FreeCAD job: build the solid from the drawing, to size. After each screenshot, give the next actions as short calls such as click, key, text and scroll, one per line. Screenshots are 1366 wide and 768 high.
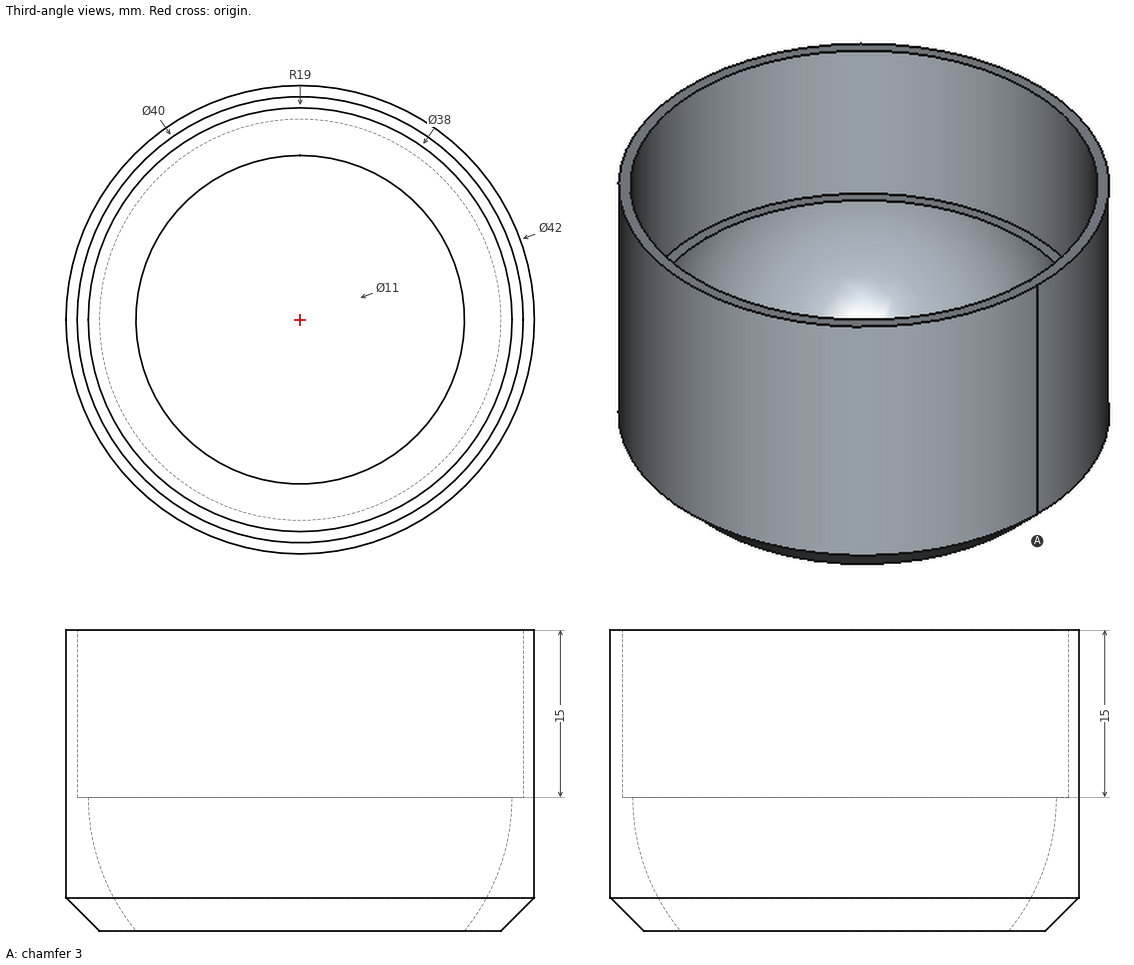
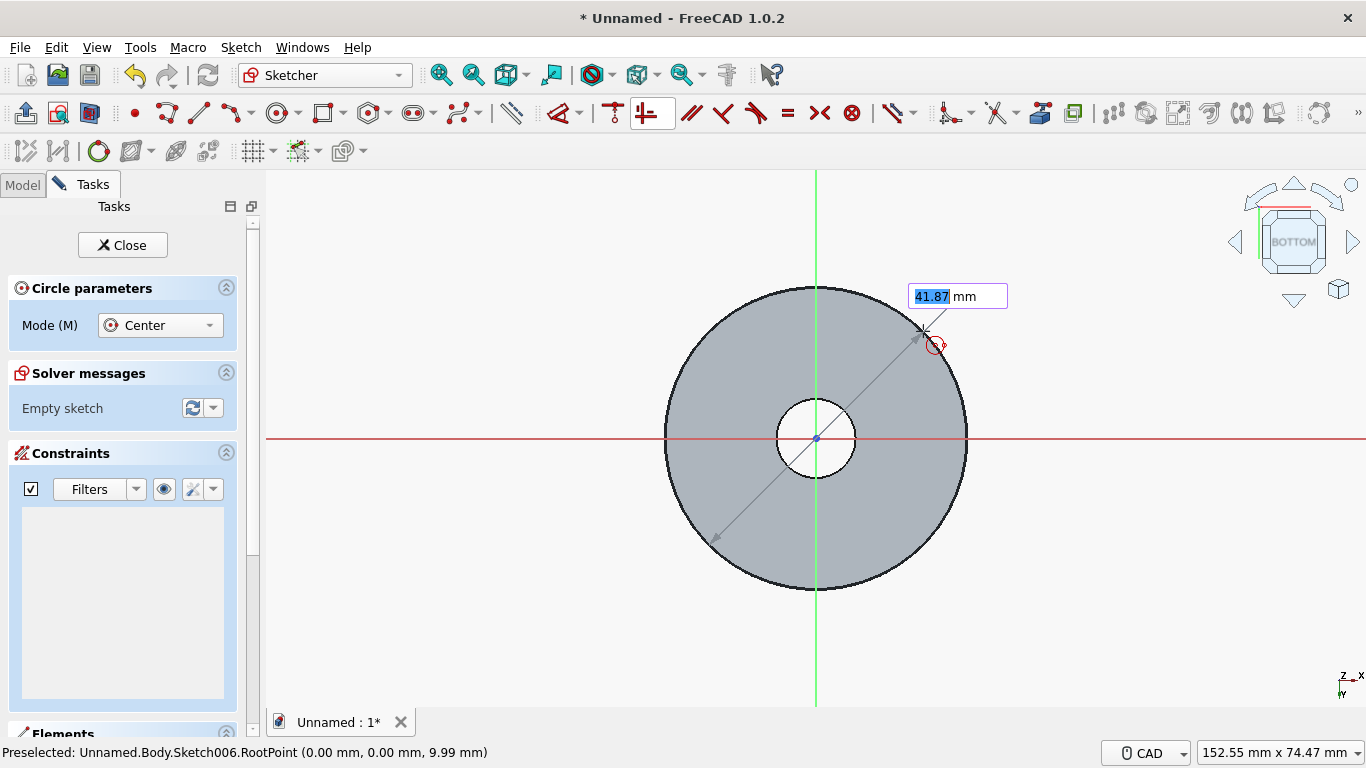
text(42)
key(Return)
key(Escape)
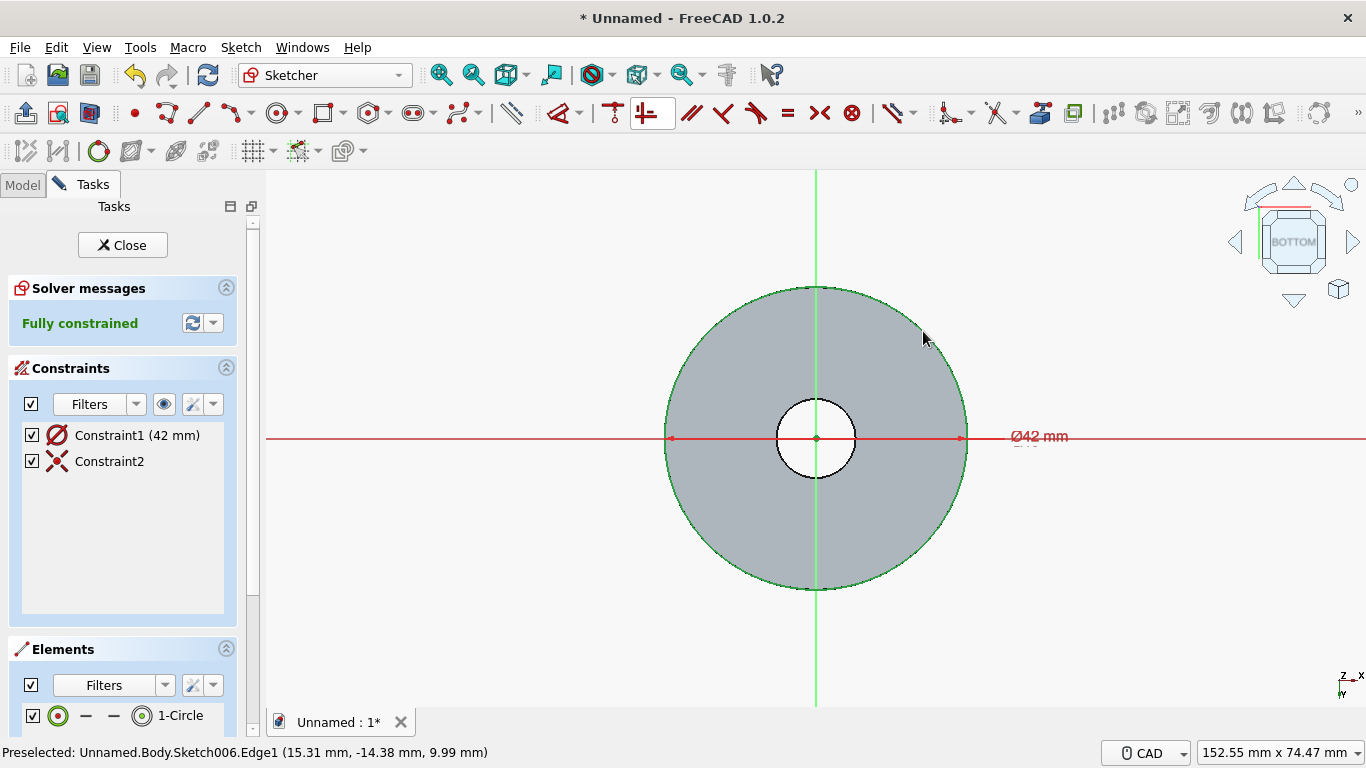
click(123, 245)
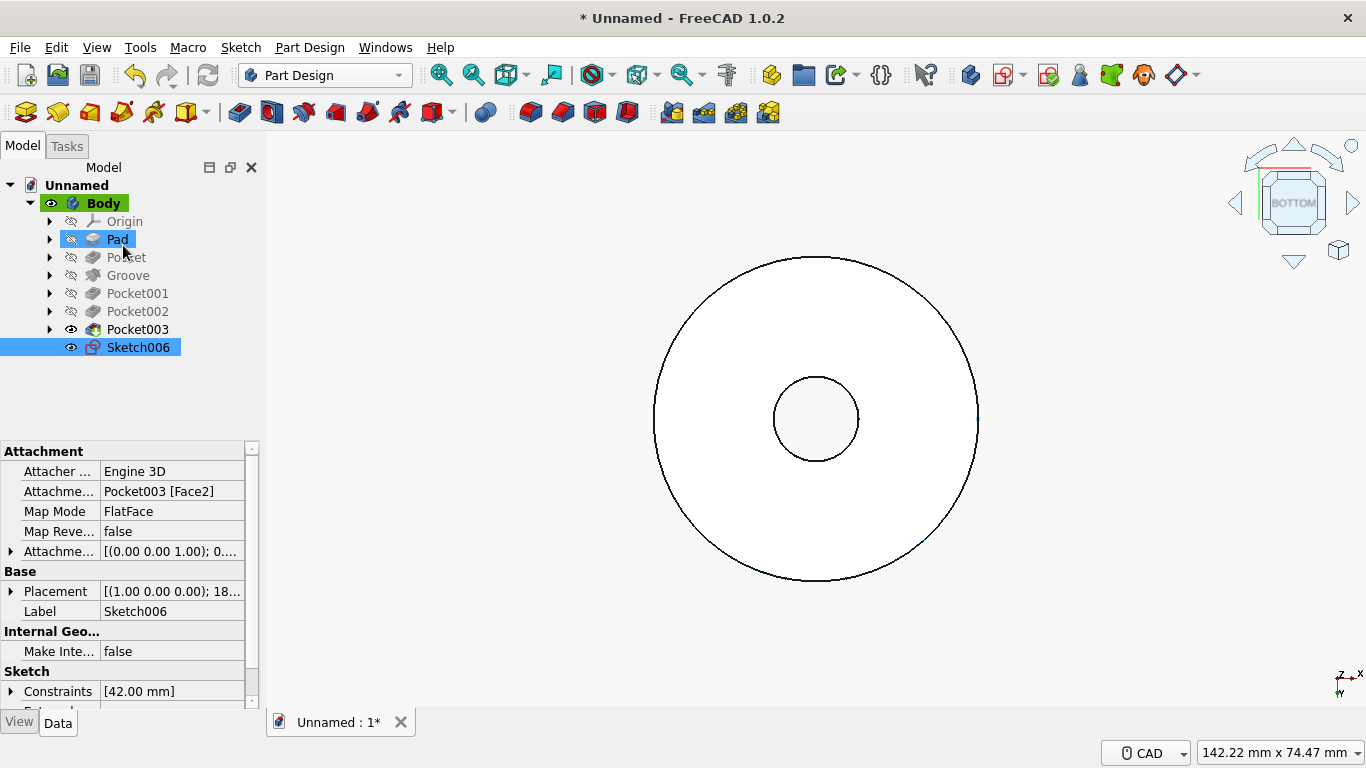
click(240, 112)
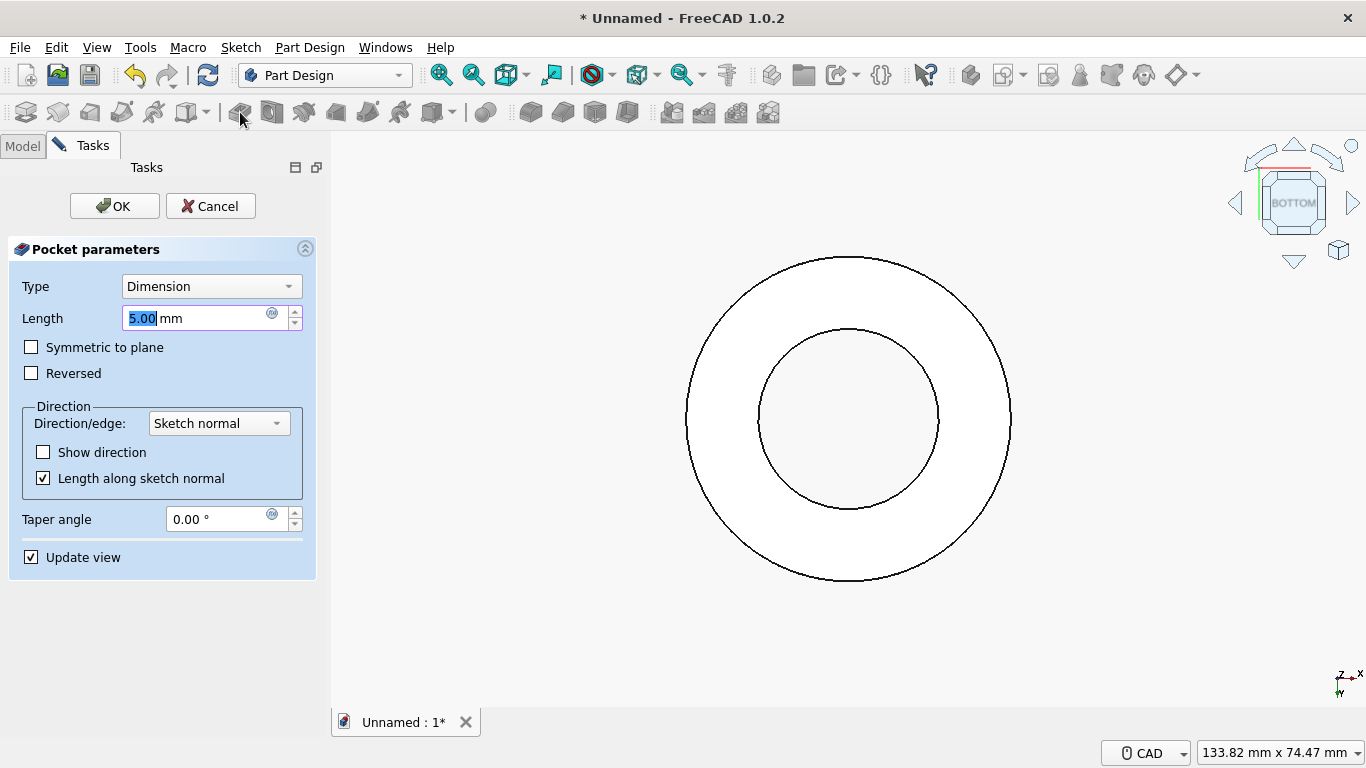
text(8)
key(Tab)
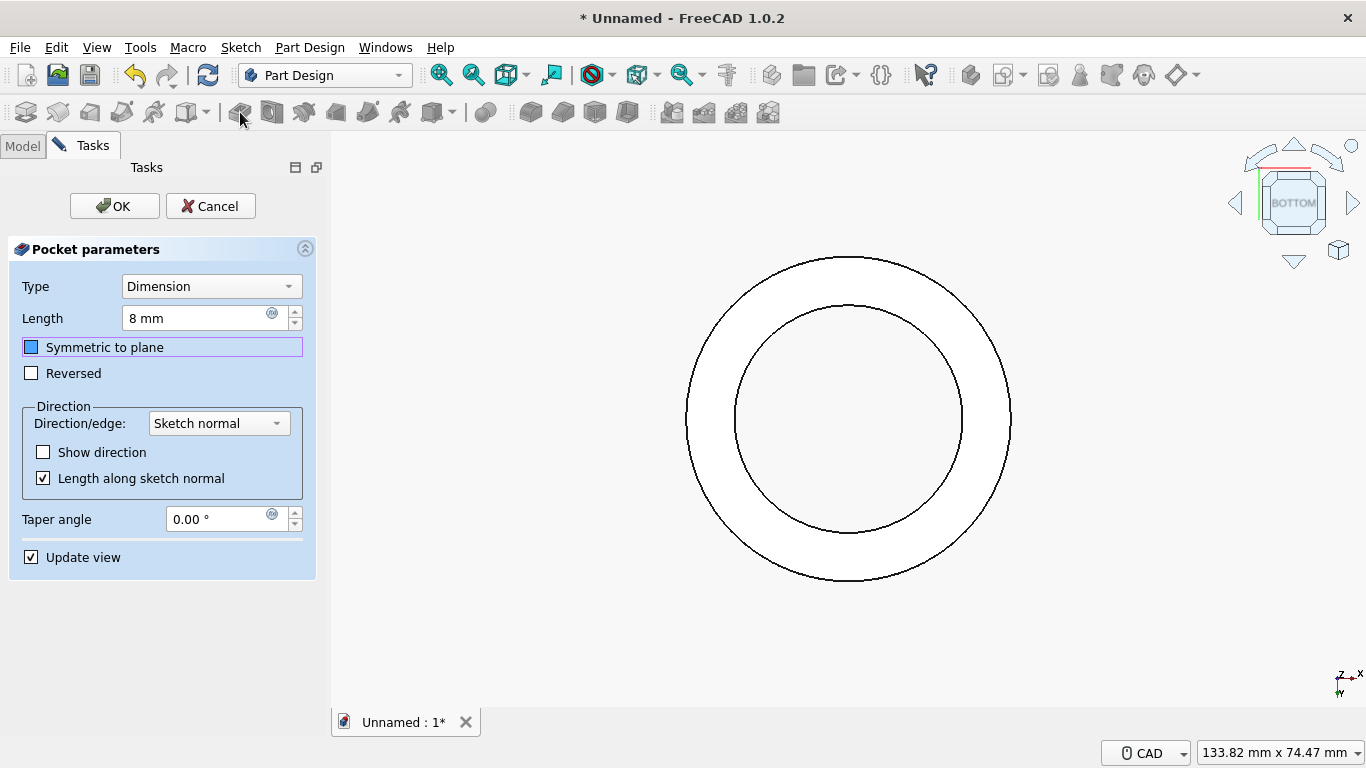
click(115, 206)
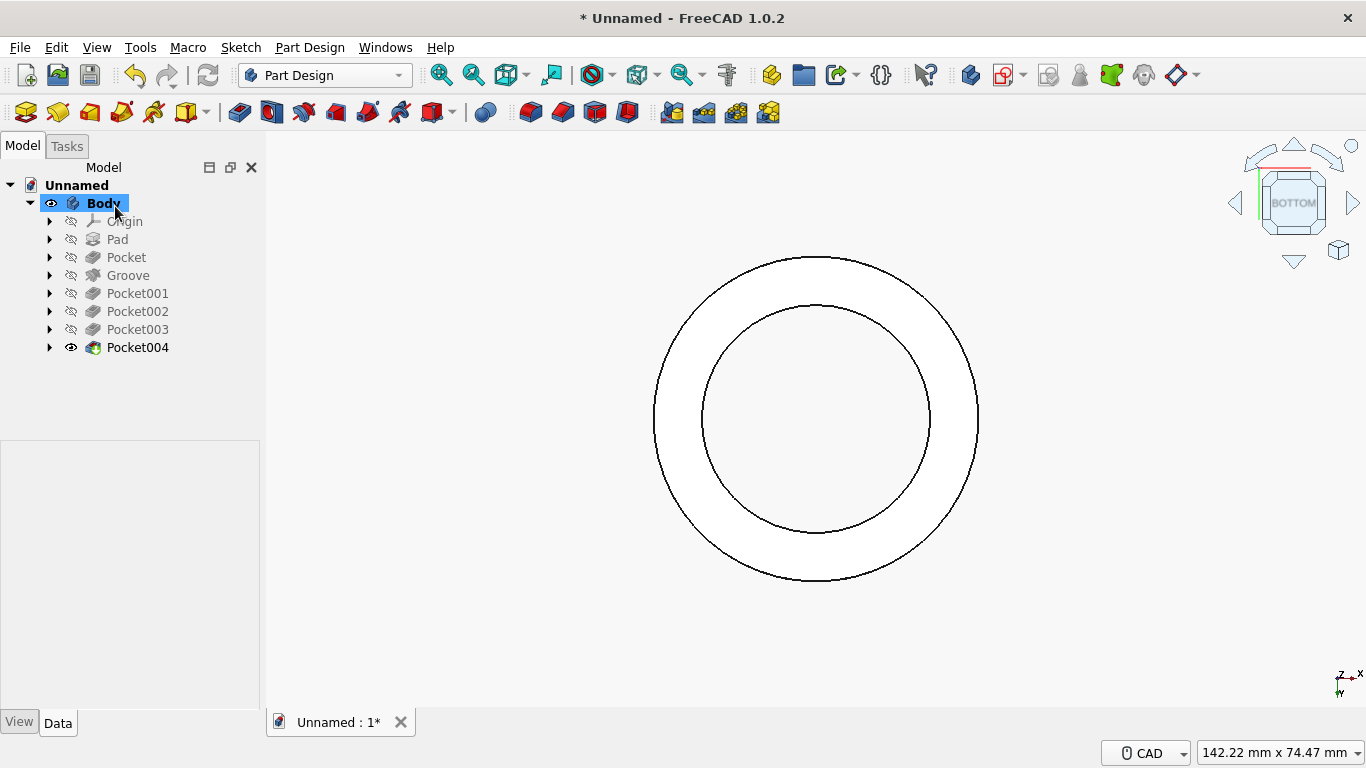
click(654, 418)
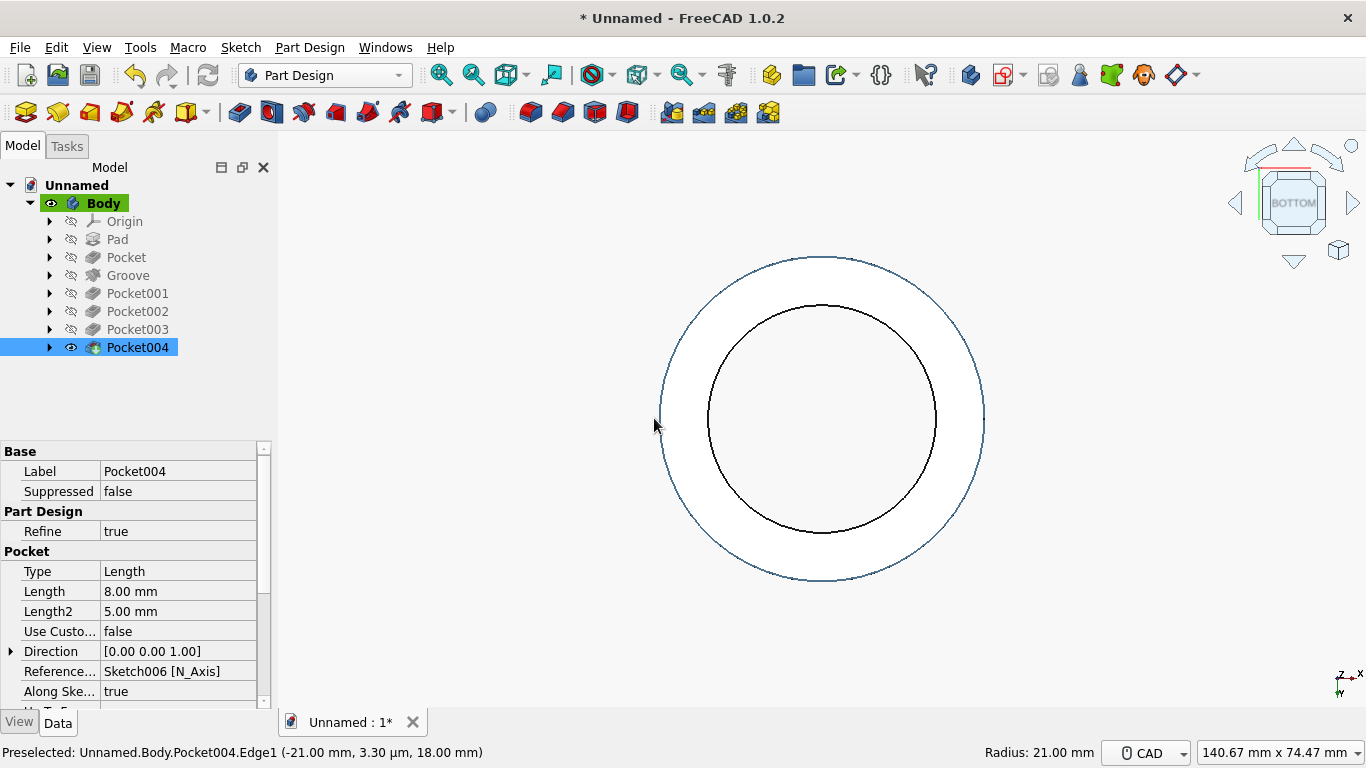
click(564, 112)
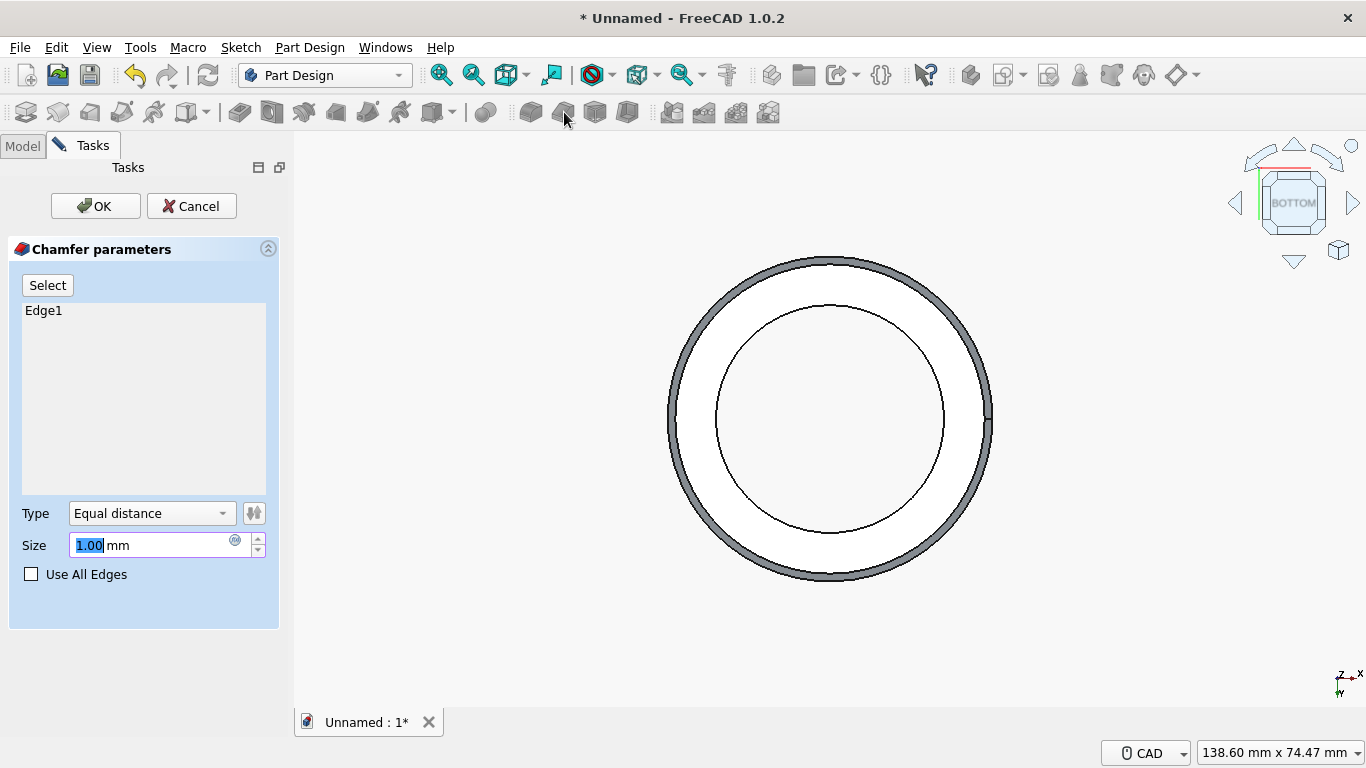
text(3)
key(Tab)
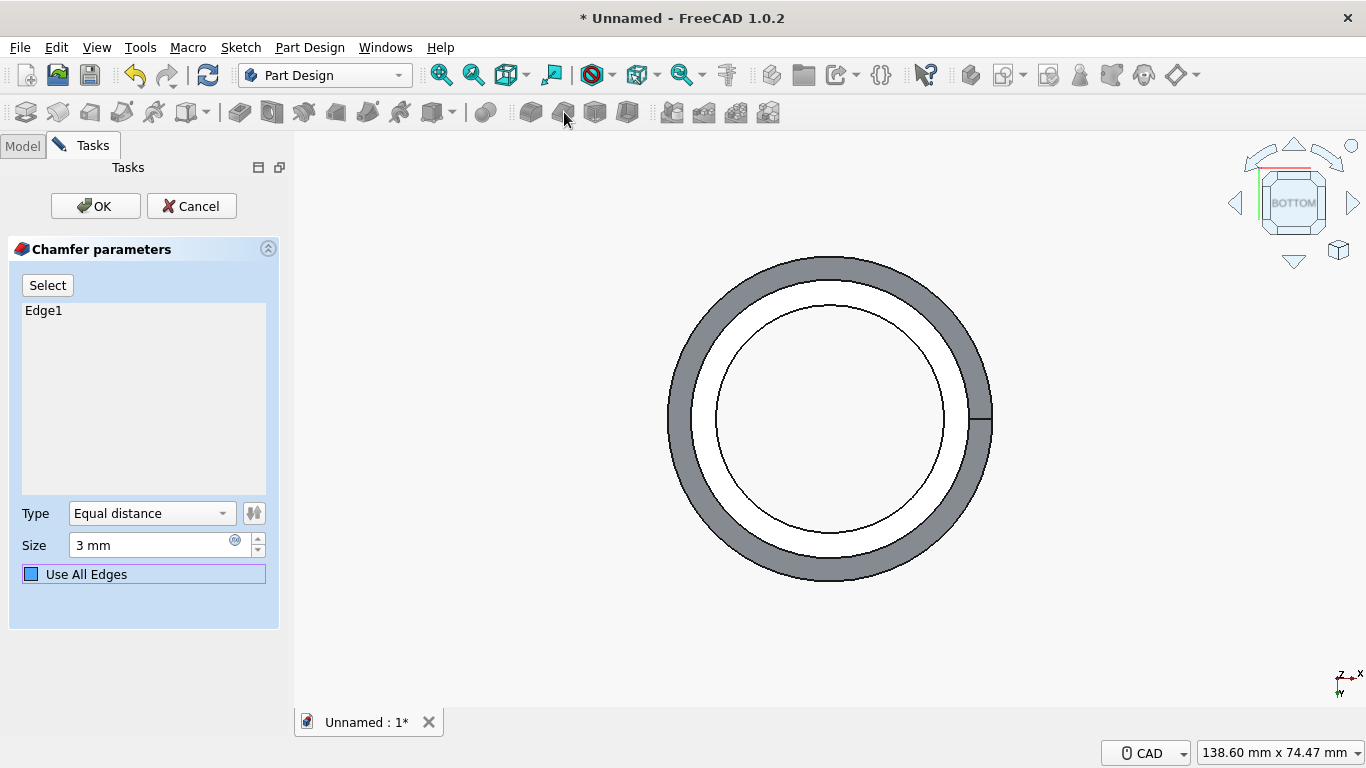
click(96, 206)